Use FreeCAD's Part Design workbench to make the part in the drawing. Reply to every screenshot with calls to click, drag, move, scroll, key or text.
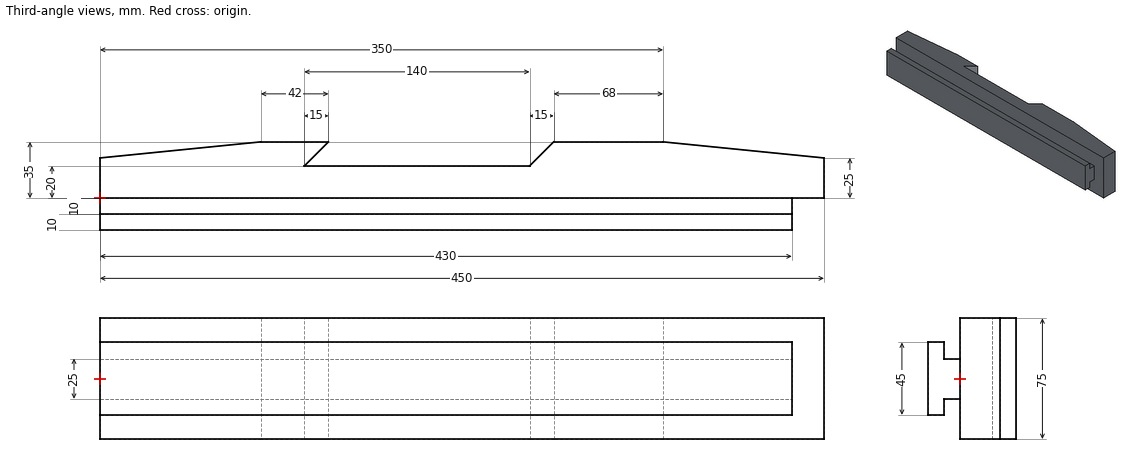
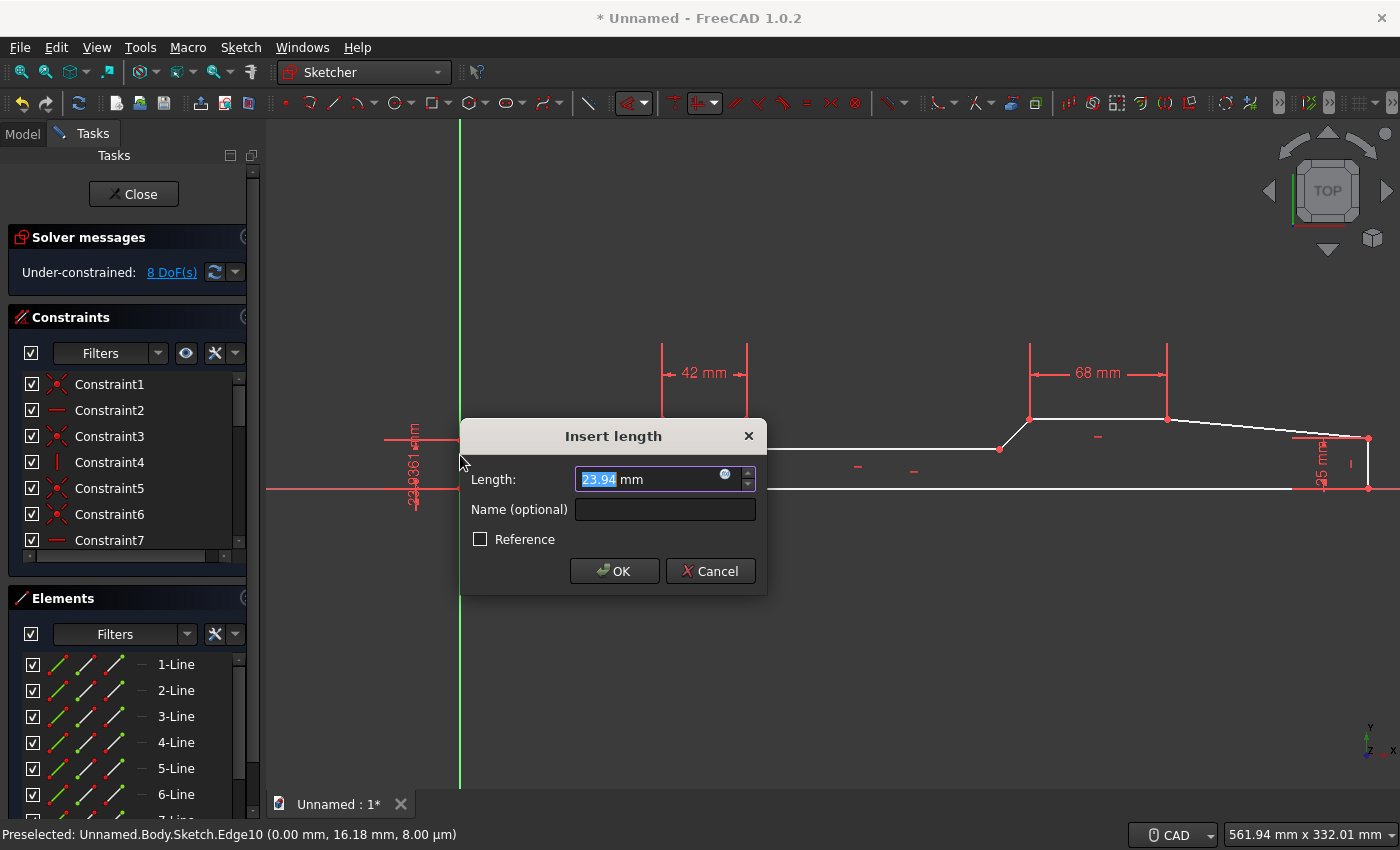
text(25)
key(Return)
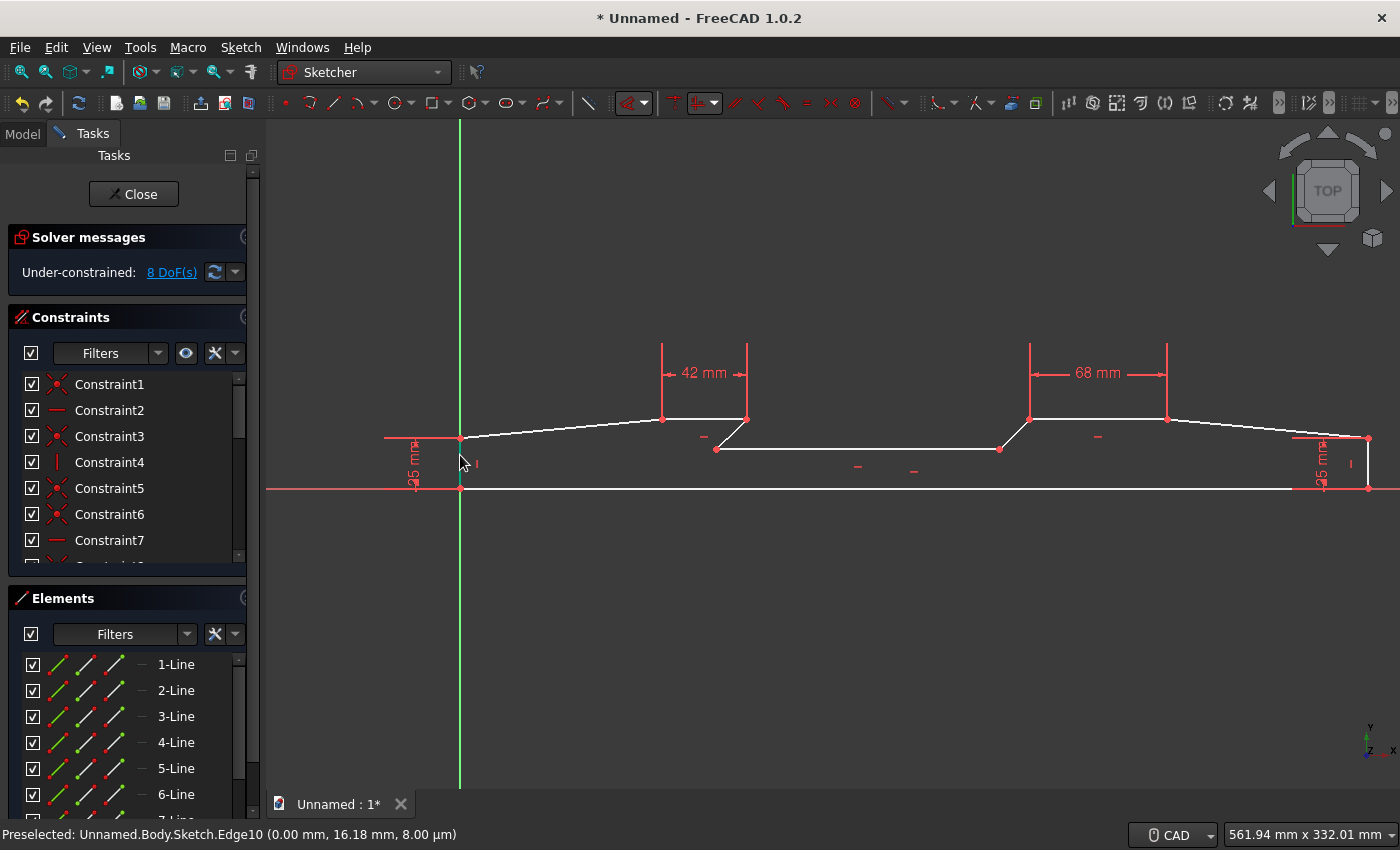
click(733, 489)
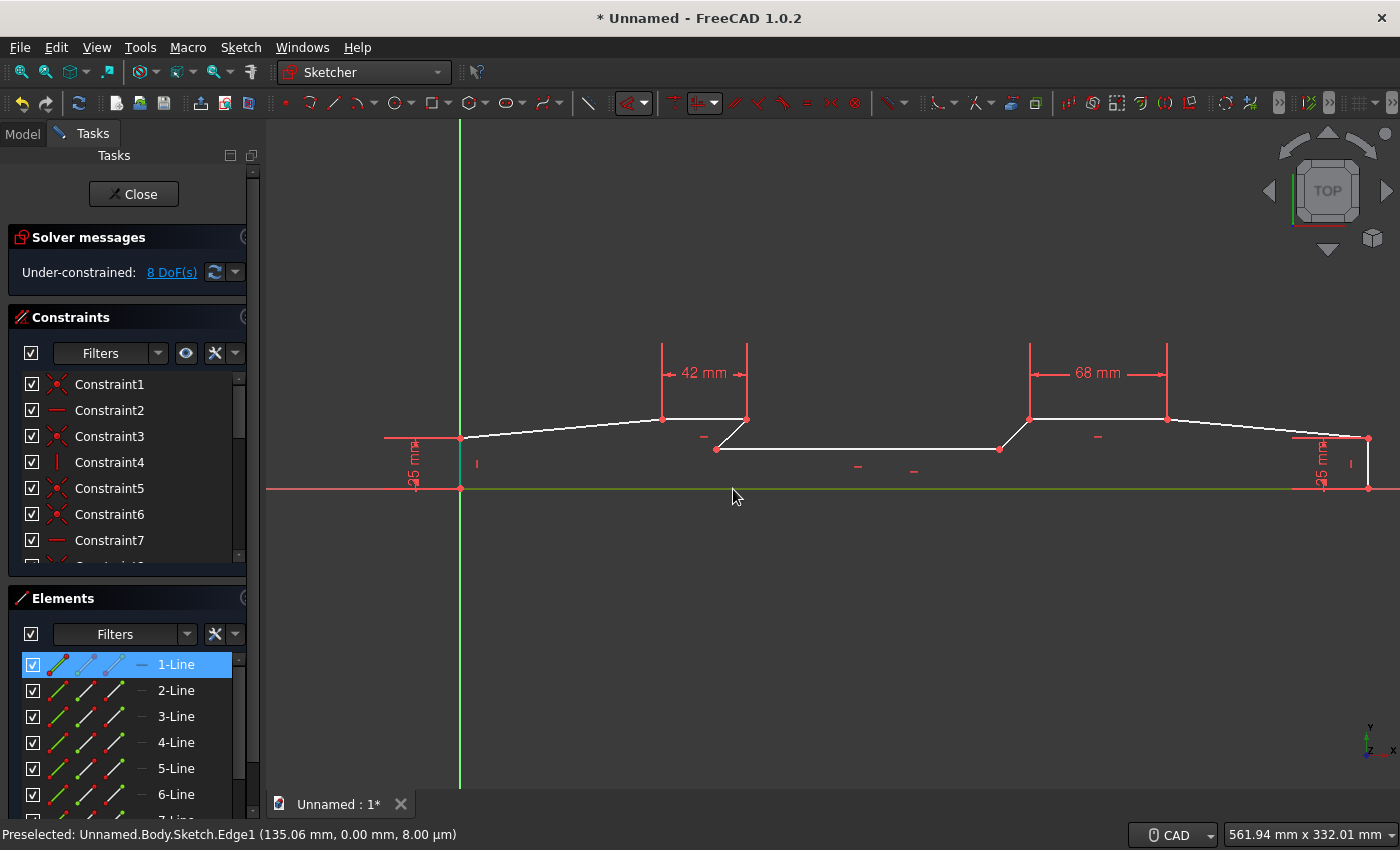
key(l)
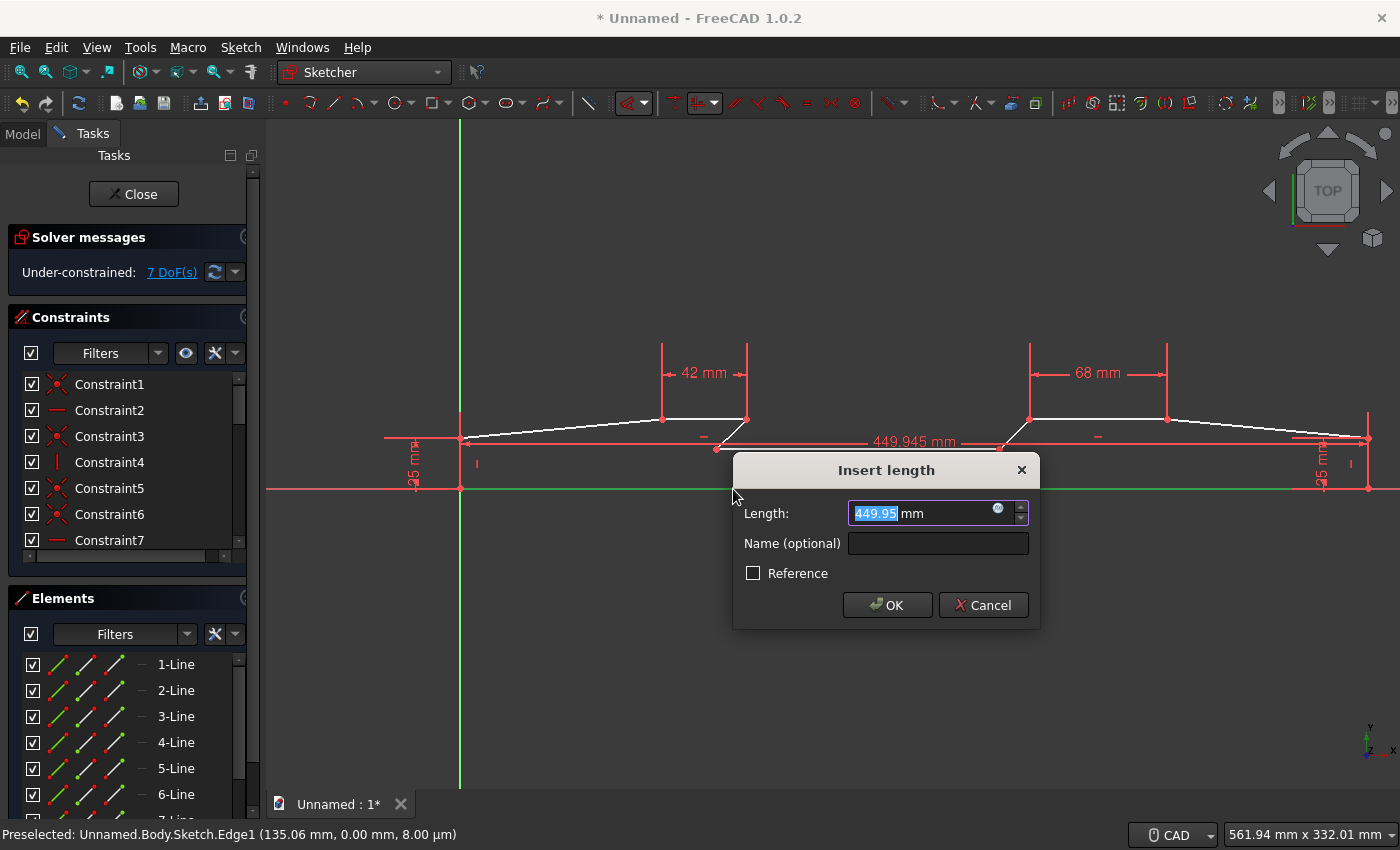
text(450)
key(Return)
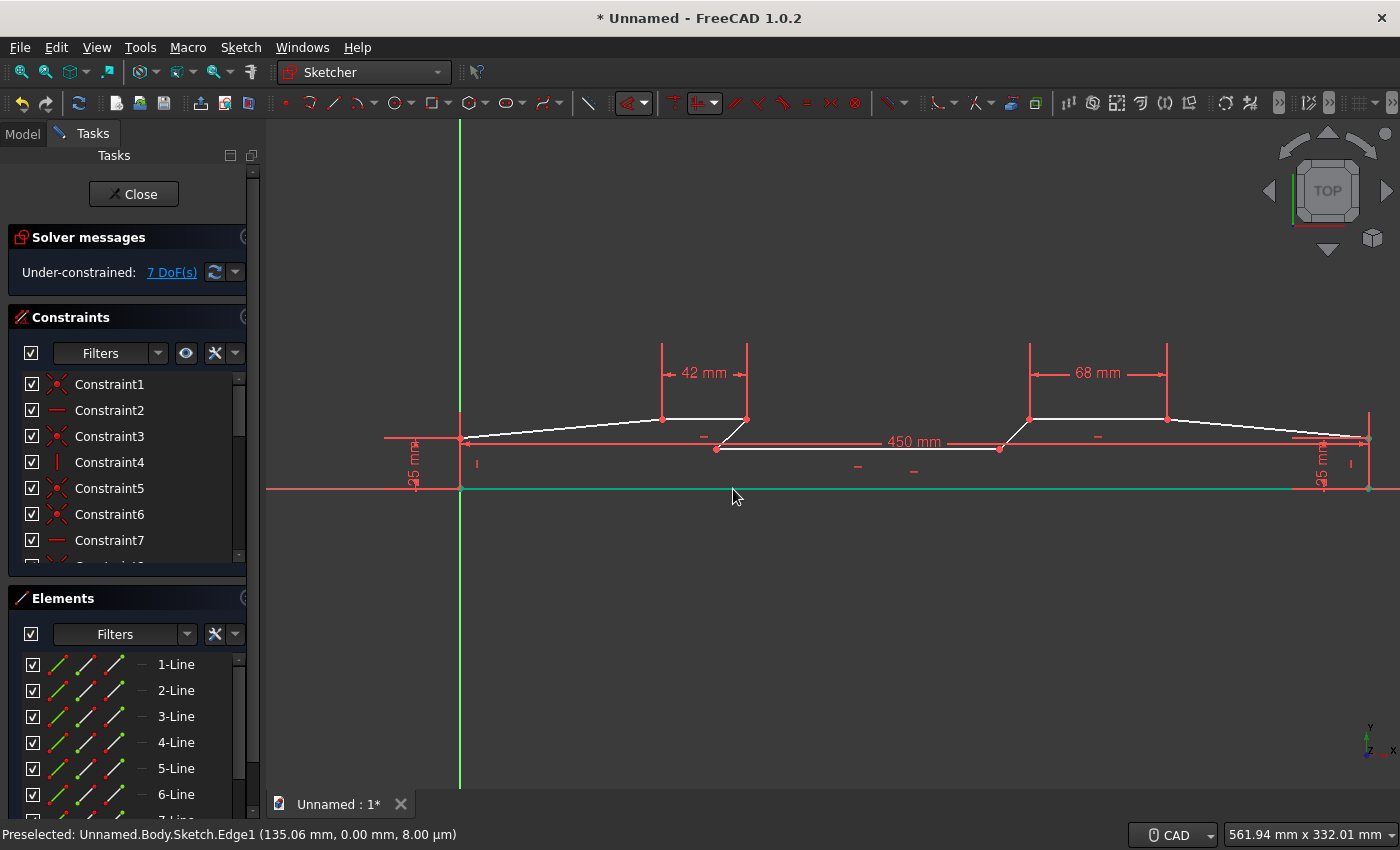
click(802, 449)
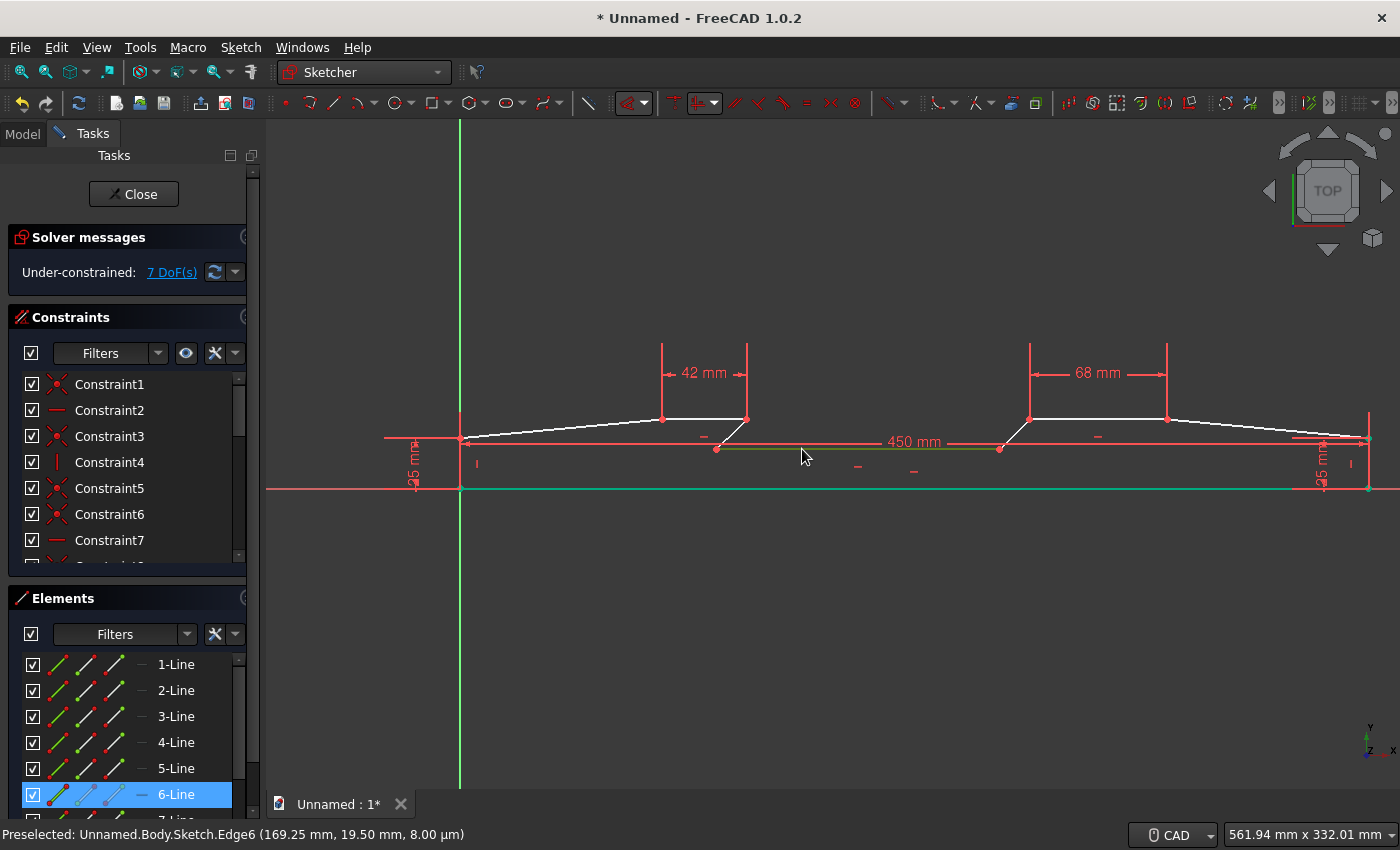
click(646, 104)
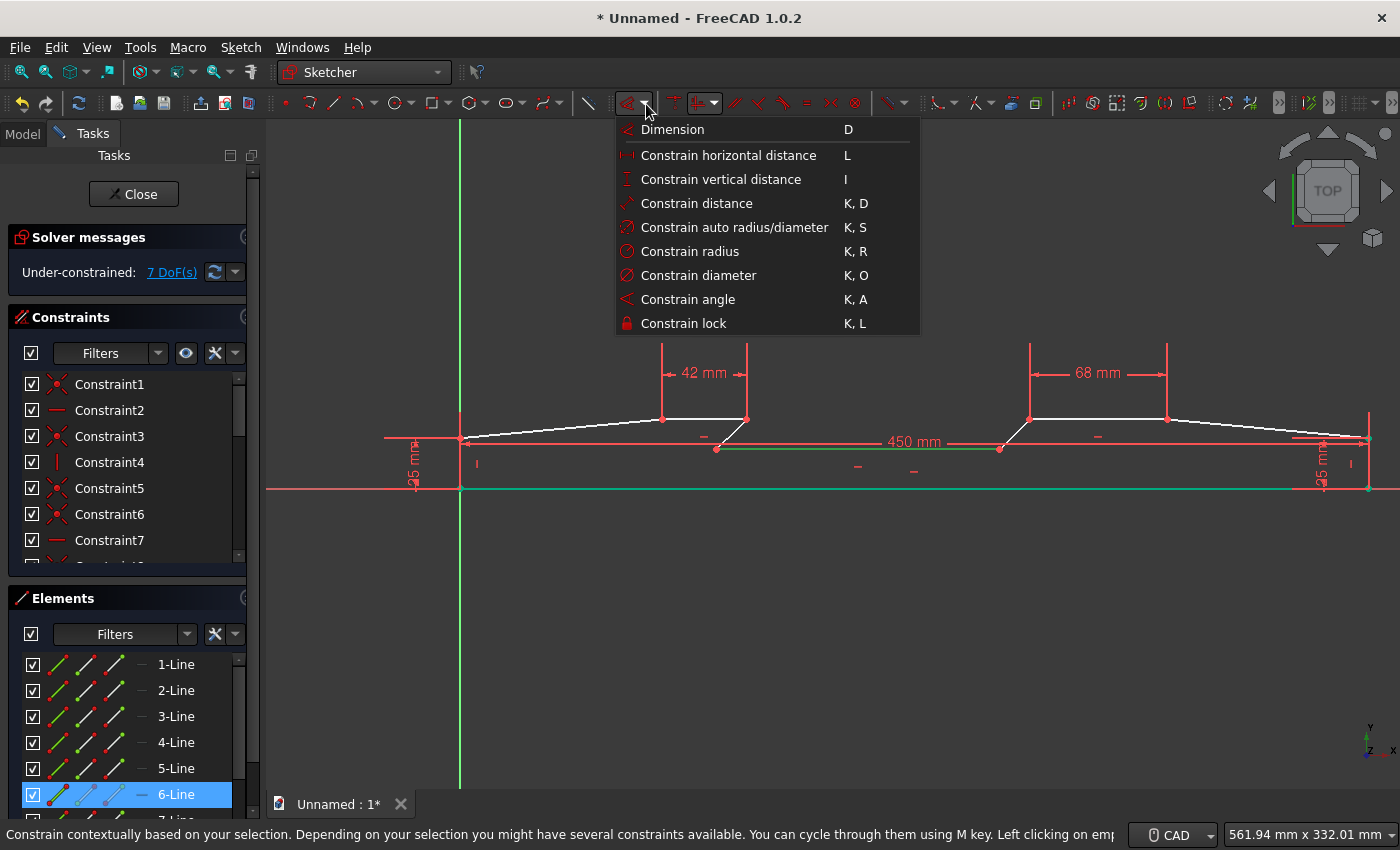
click(768, 155)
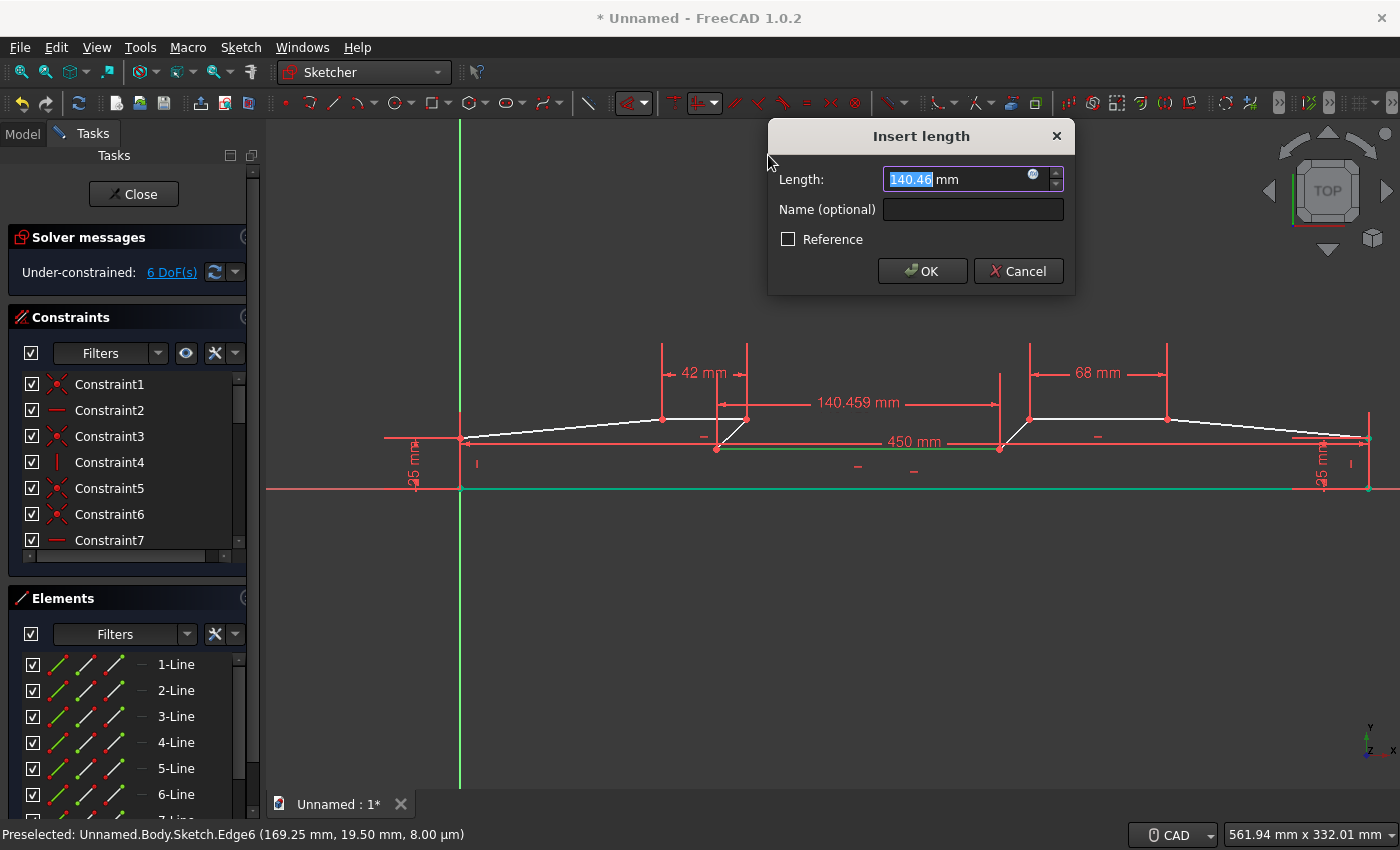
text(140)
key(Return)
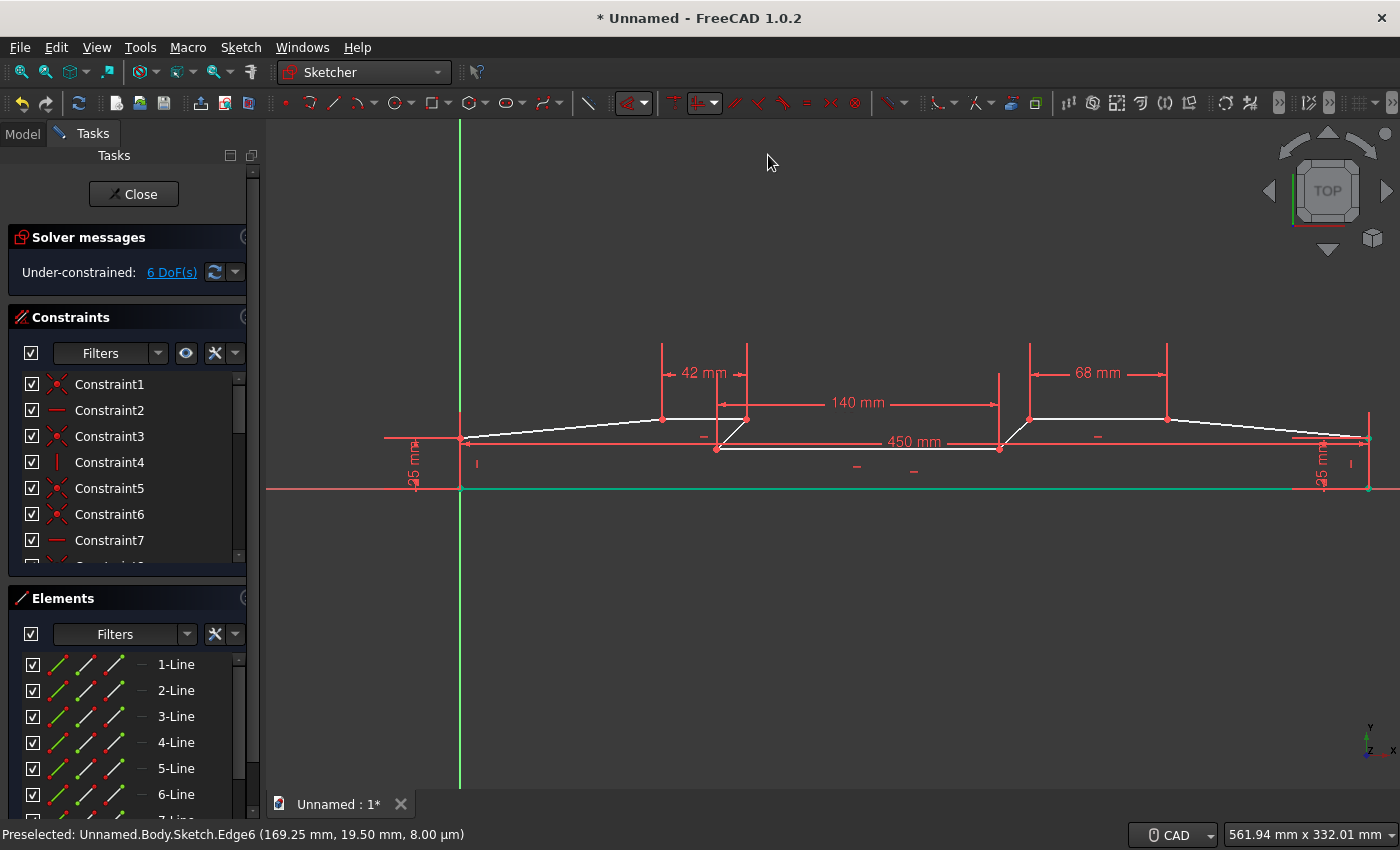
click(1167, 419)